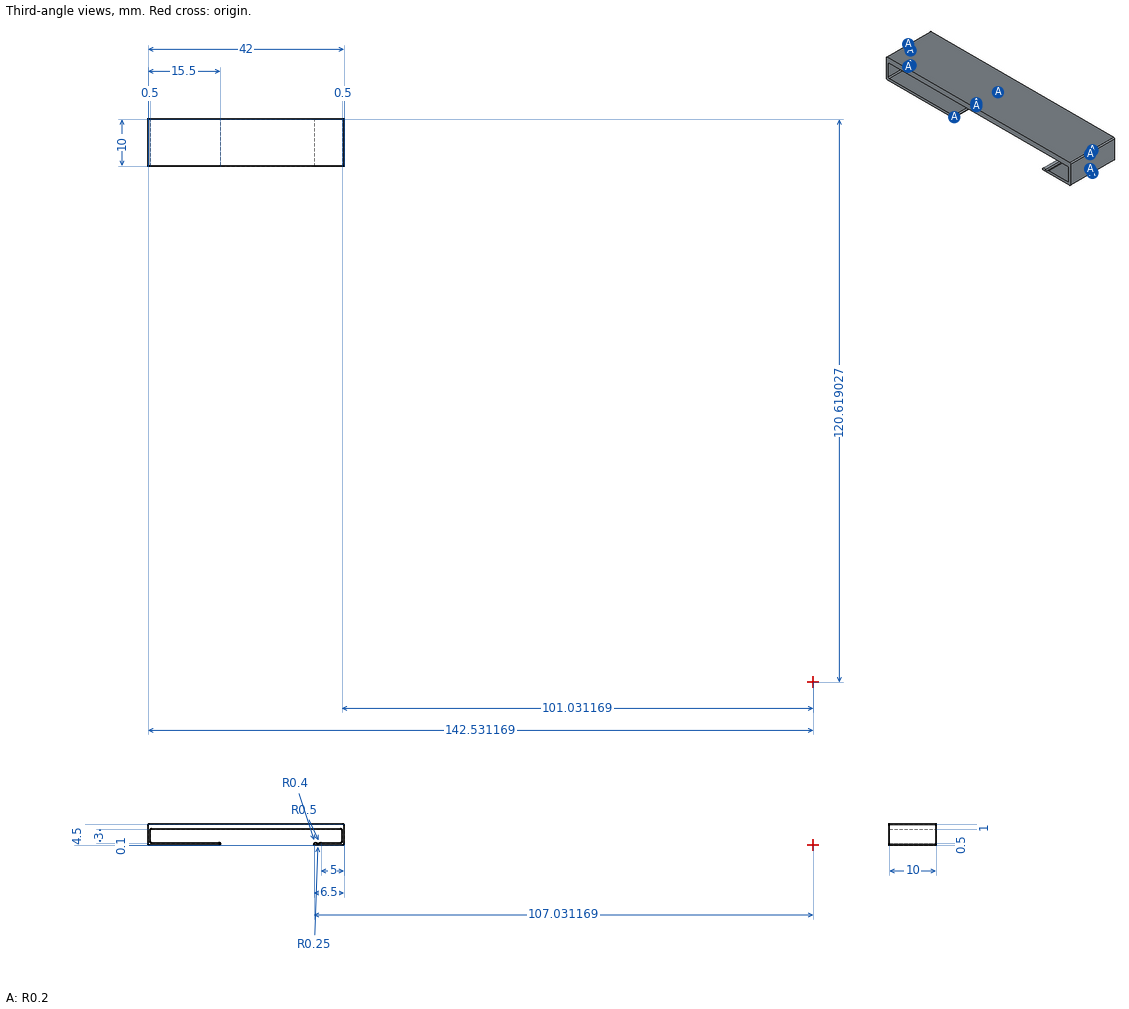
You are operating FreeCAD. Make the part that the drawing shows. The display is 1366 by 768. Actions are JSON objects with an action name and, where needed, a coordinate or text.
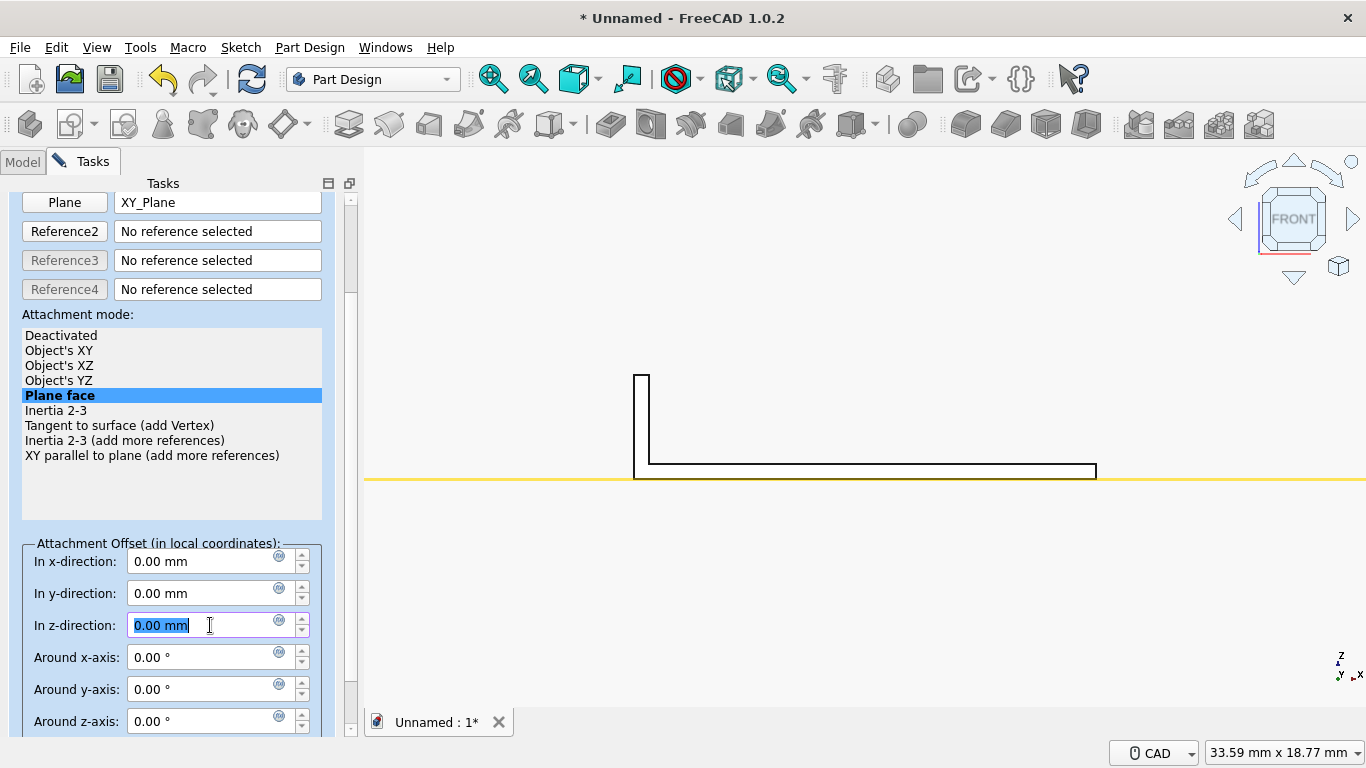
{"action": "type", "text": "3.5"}
{"action": "key", "text": "Tab"}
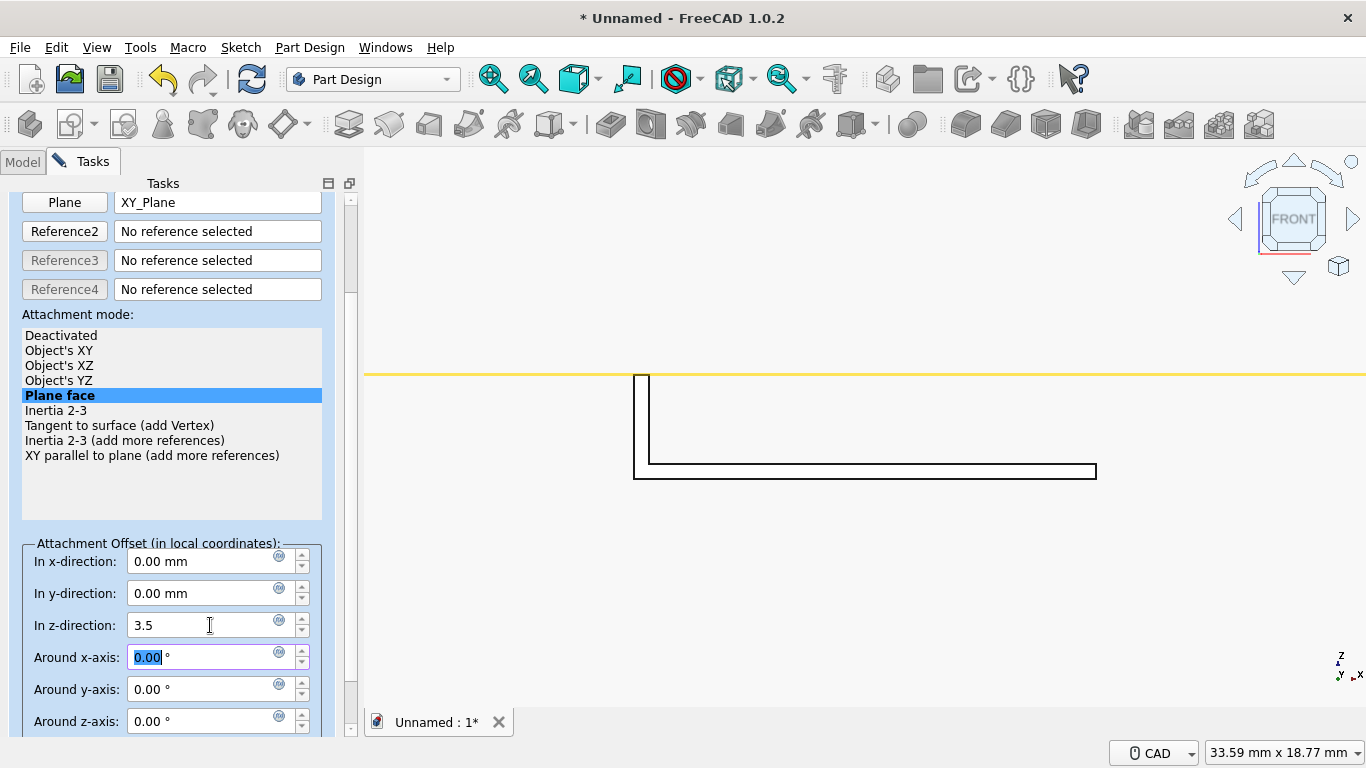
{"action": "scroll", "coordinate": [351, 464], "scroll_direction": "up", "scroll_amount": 3}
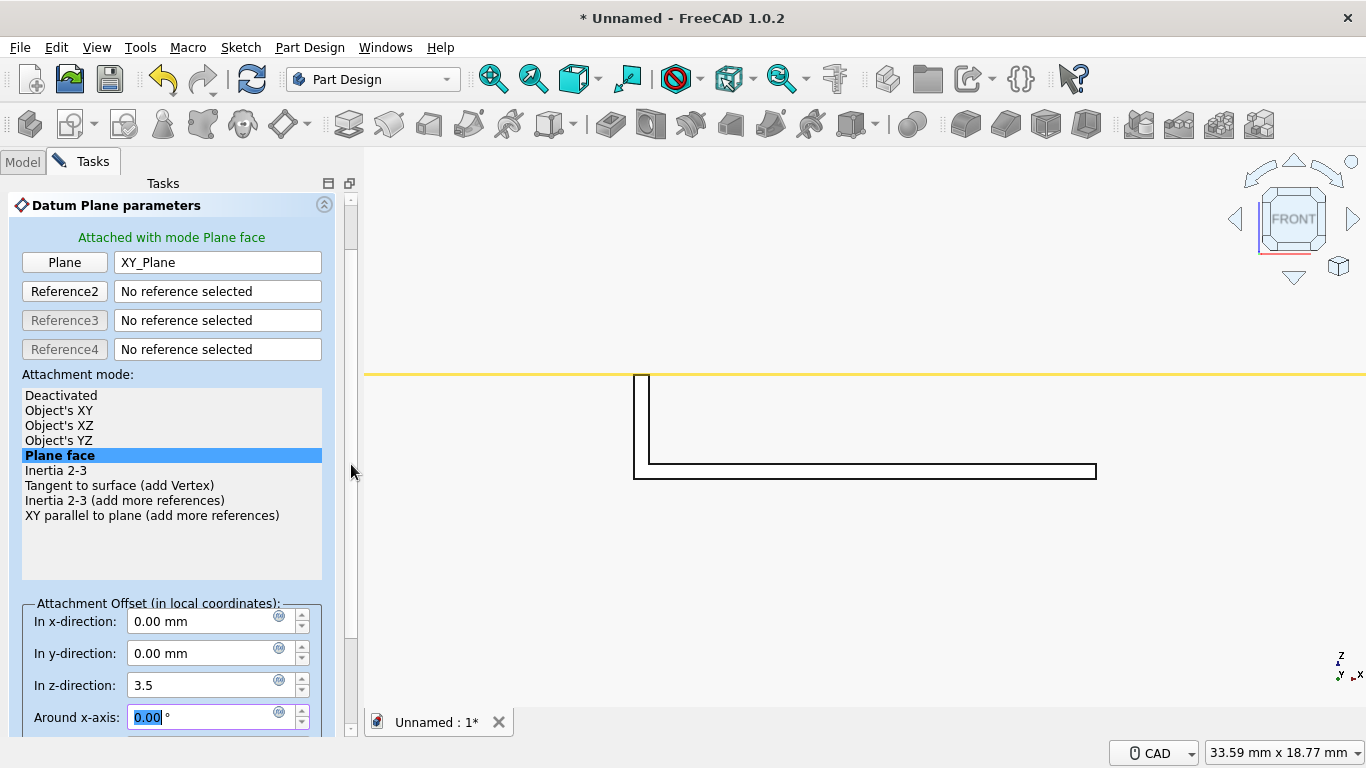
{"action": "left_click", "coordinate": [124, 222]}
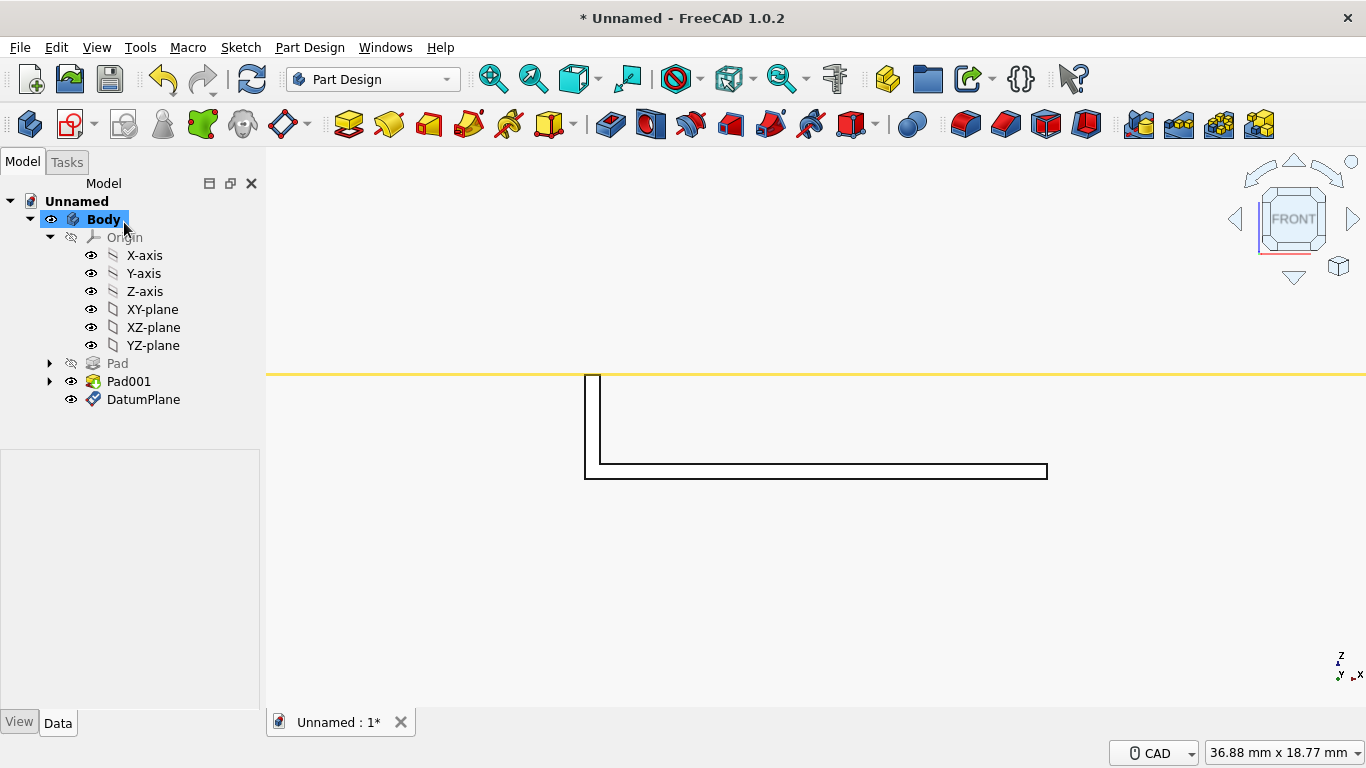
{"action": "left_click", "coordinate": [116, 399]}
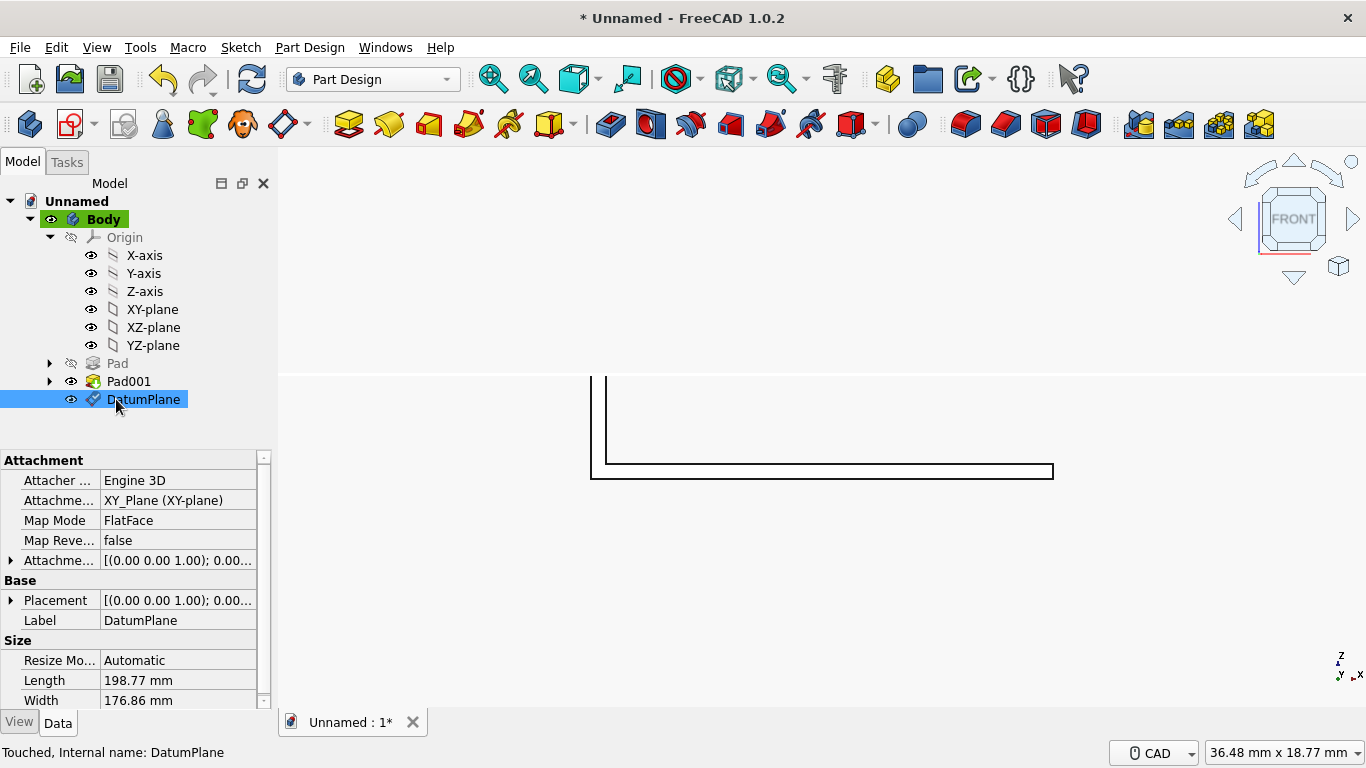
{"action": "left_click", "coordinate": [70, 124]}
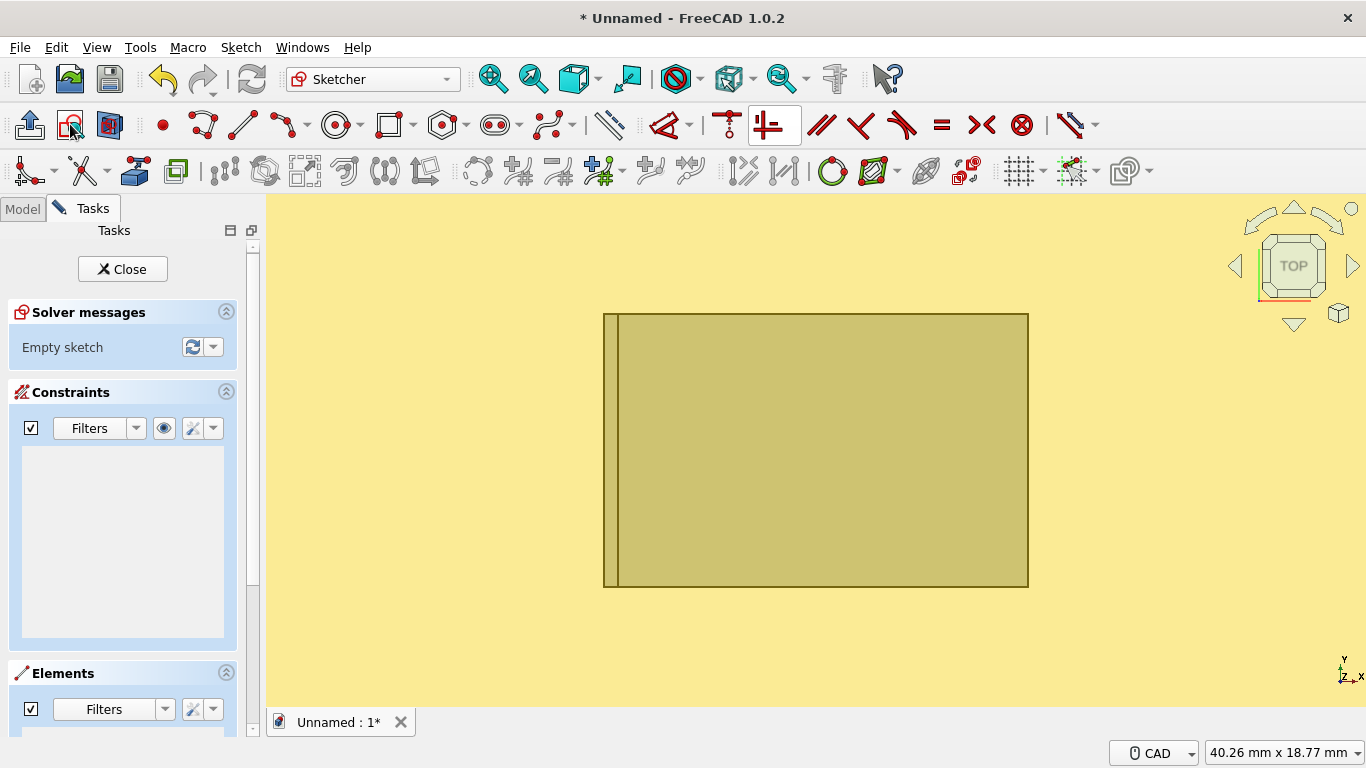
{"action": "scroll", "coordinate": [294, 451], "scroll_direction": "down", "scroll_amount": 3}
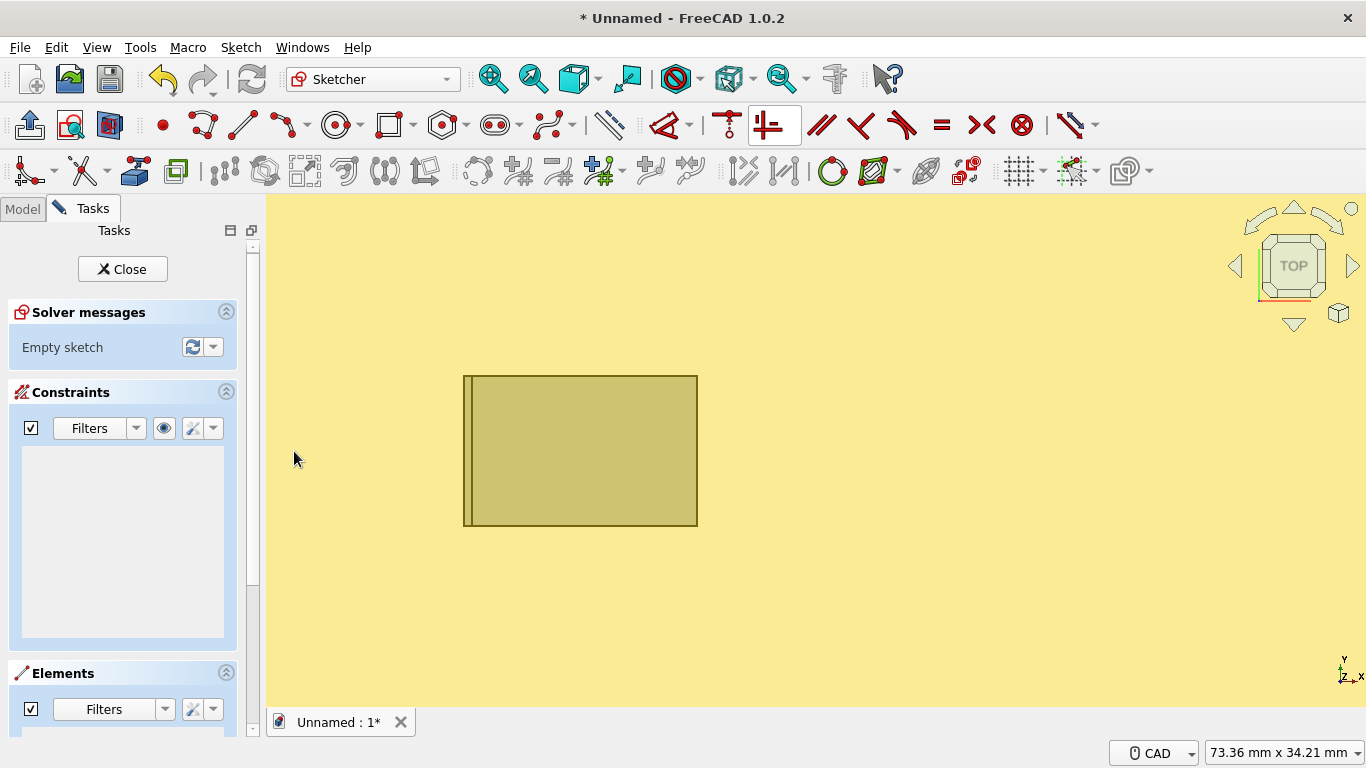
{"action": "left_click", "coordinate": [390, 126]}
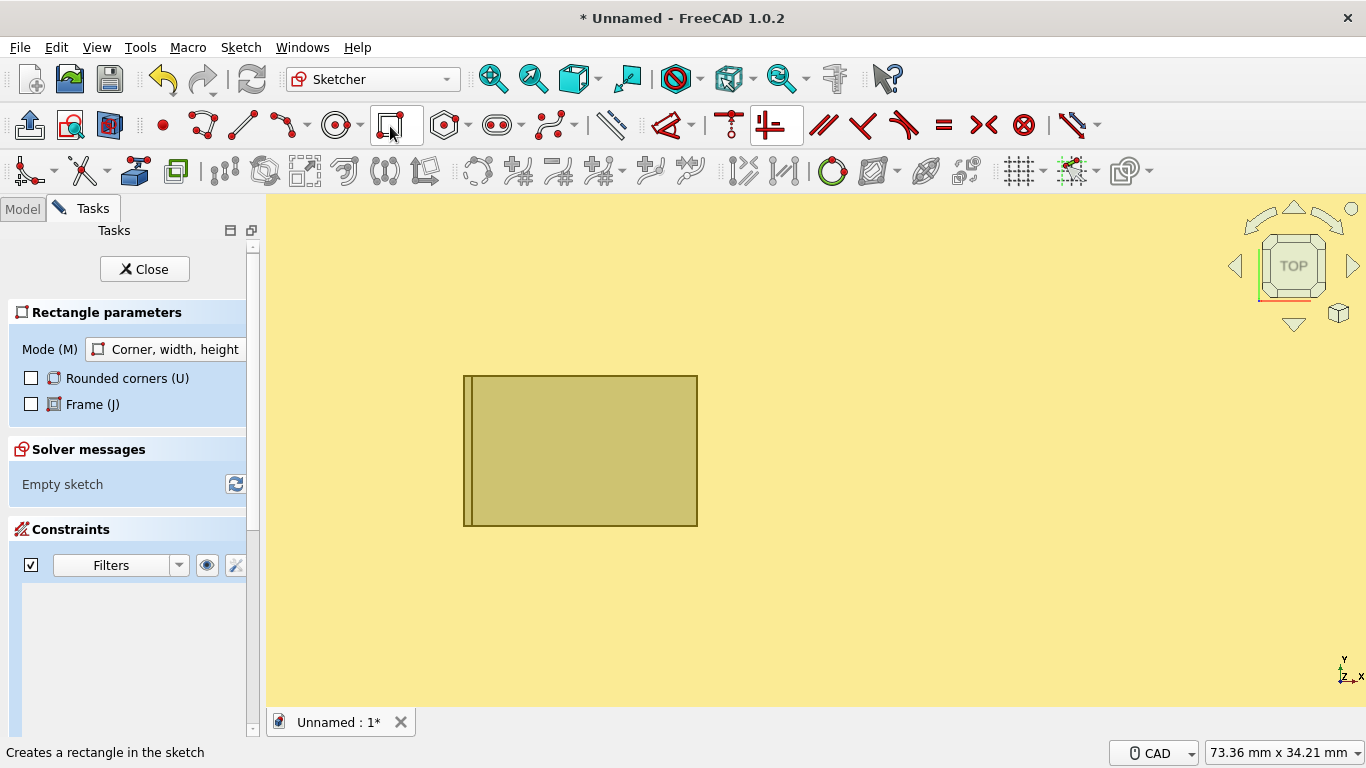
{"action": "left_click", "coordinate": [464, 376]}
{"action": "left_click", "coordinate": [1094, 526]}
{"action": "key", "text": "Escape"}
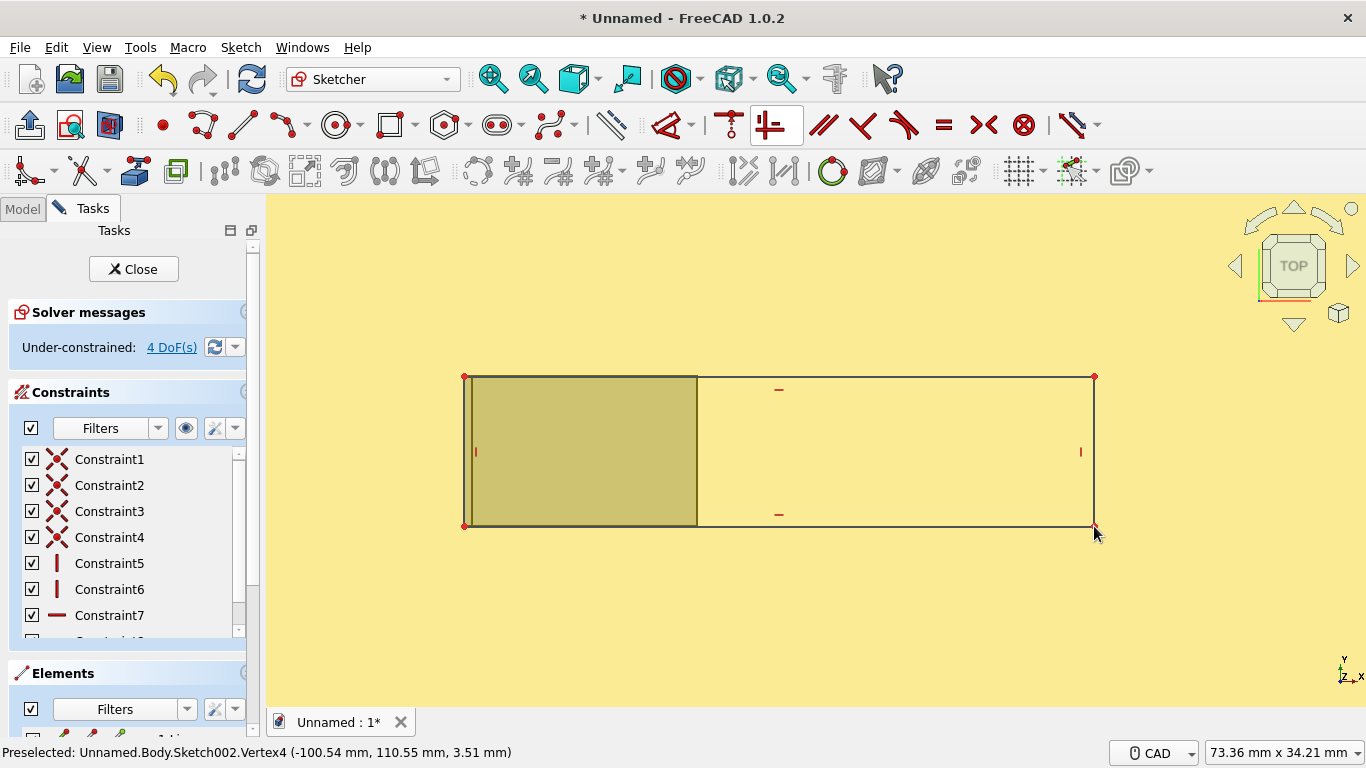
{"action": "left_click", "coordinate": [666, 126]}